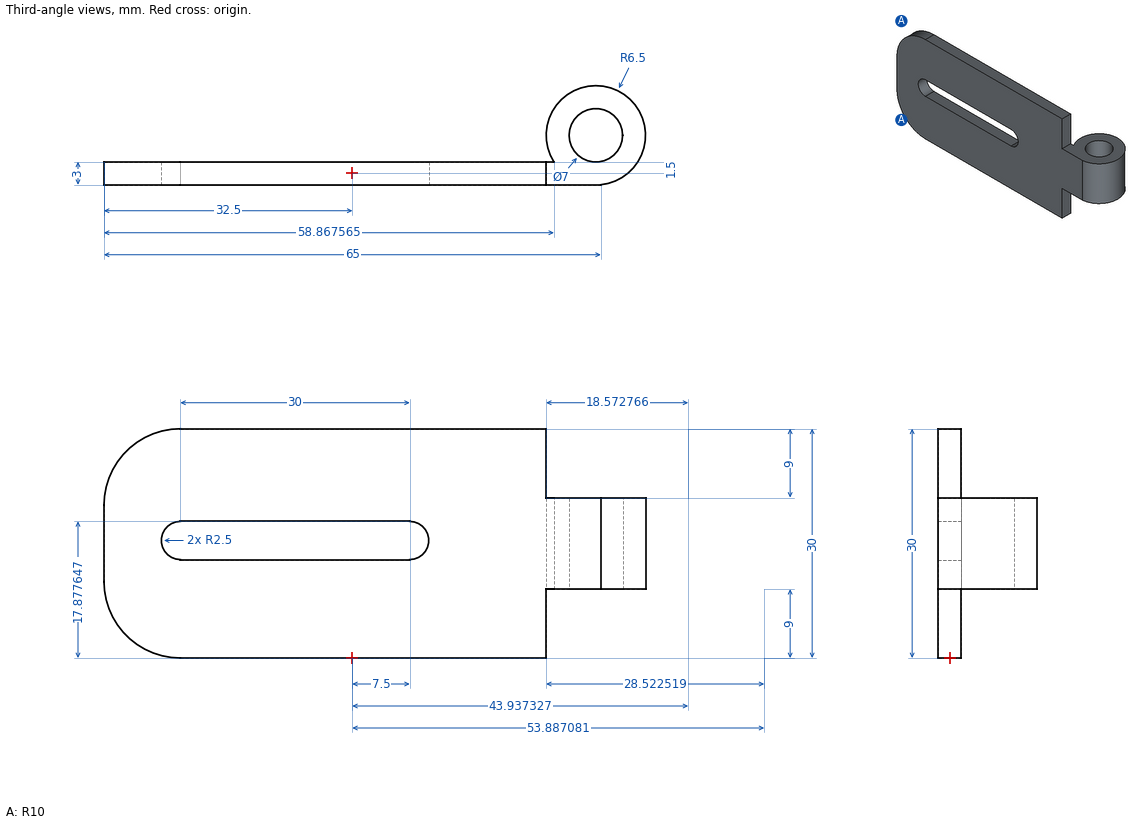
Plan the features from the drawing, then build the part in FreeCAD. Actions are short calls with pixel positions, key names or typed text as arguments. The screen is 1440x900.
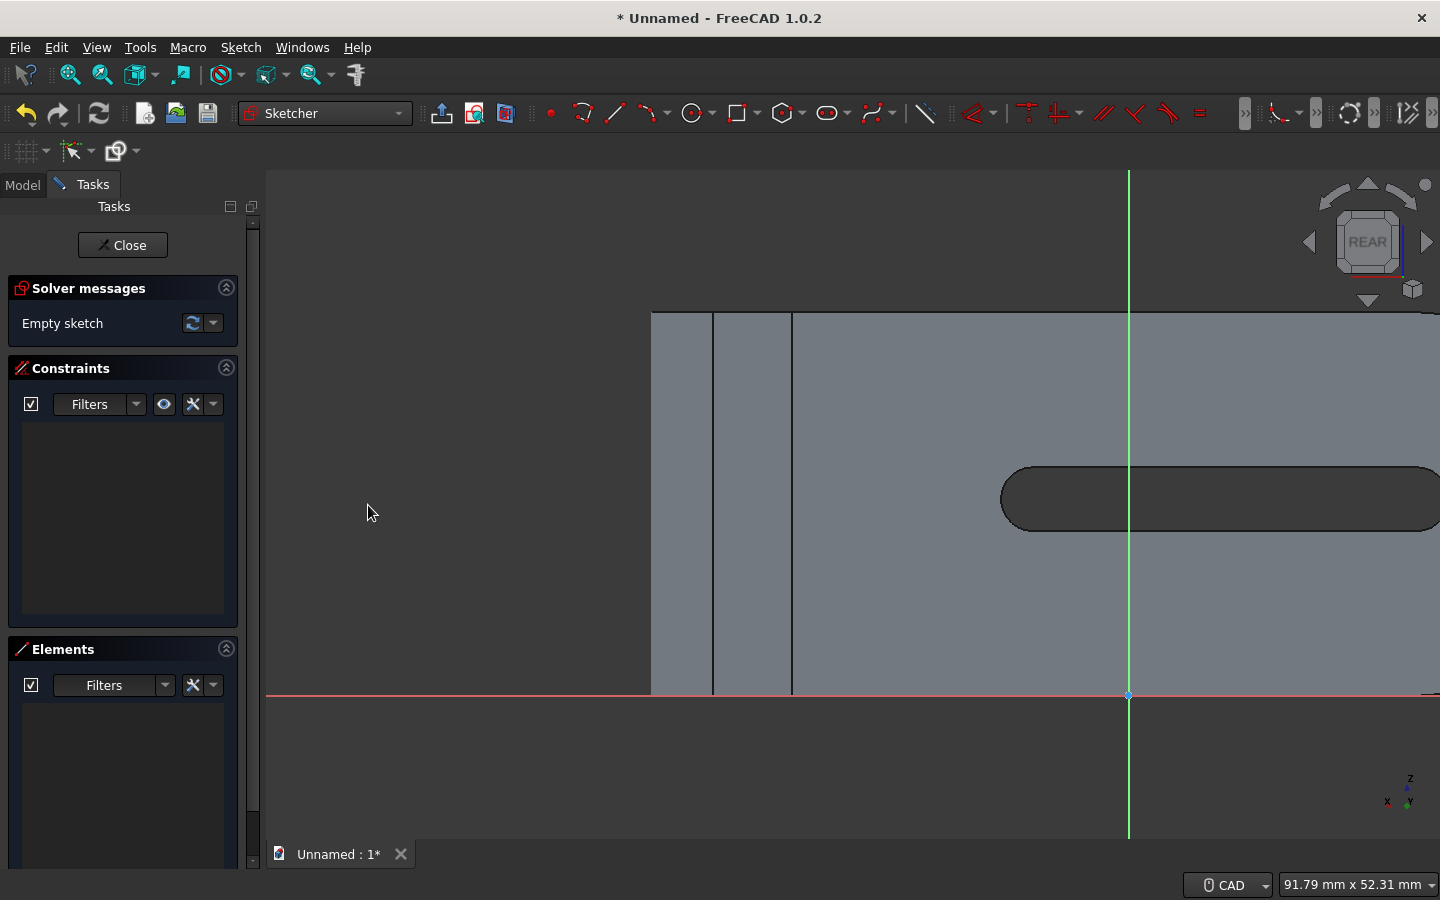
click(738, 114)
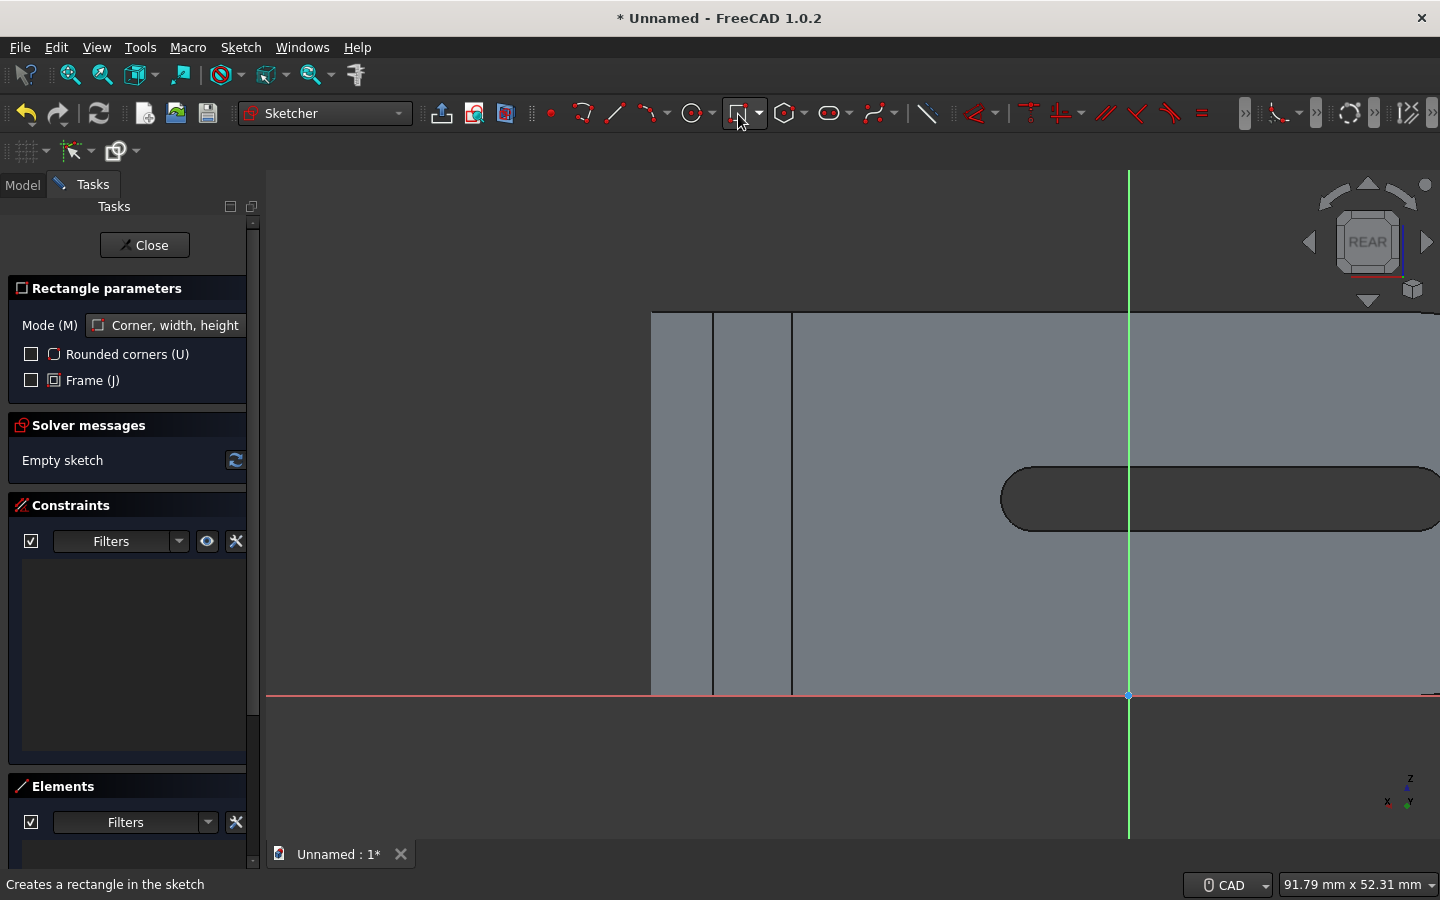
click(567, 312)
move(805, 427)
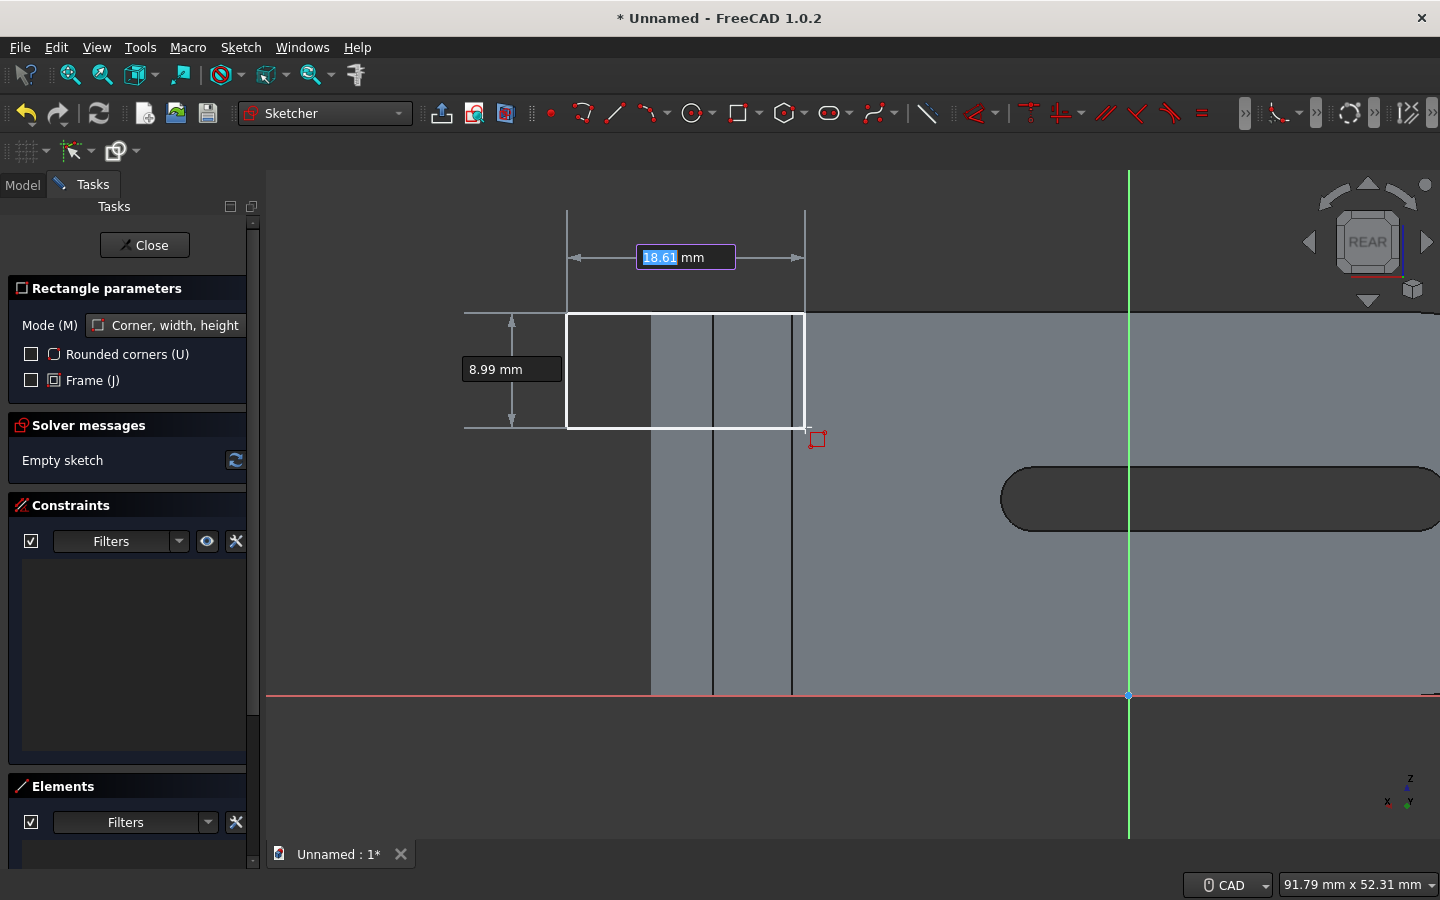
text(18.572766)
key(Tab)
text(9)
key(Return)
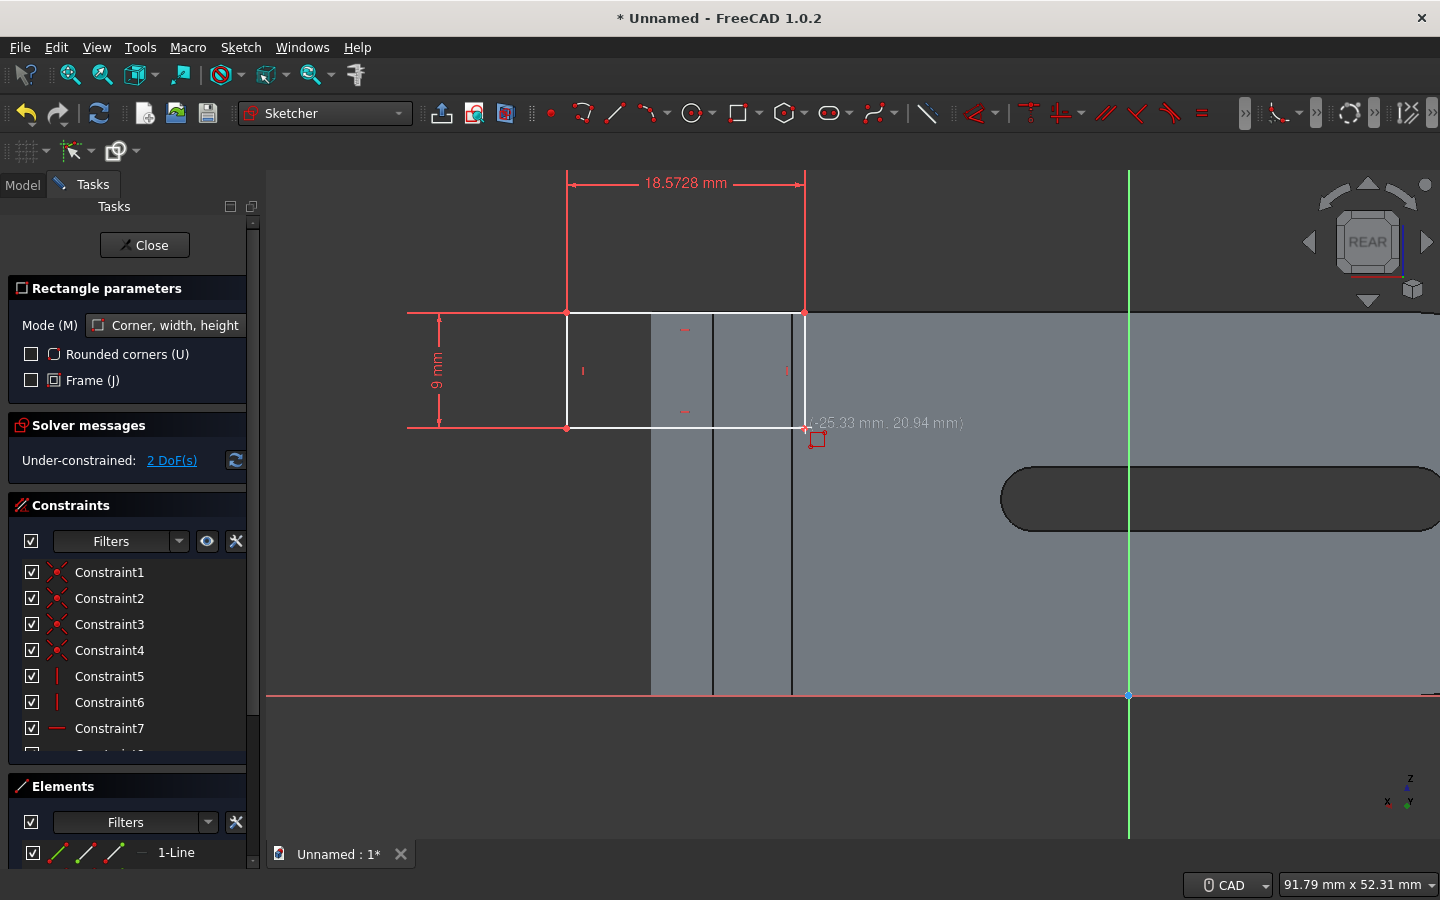
click(440, 581)
click(805, 696)
key(Escape)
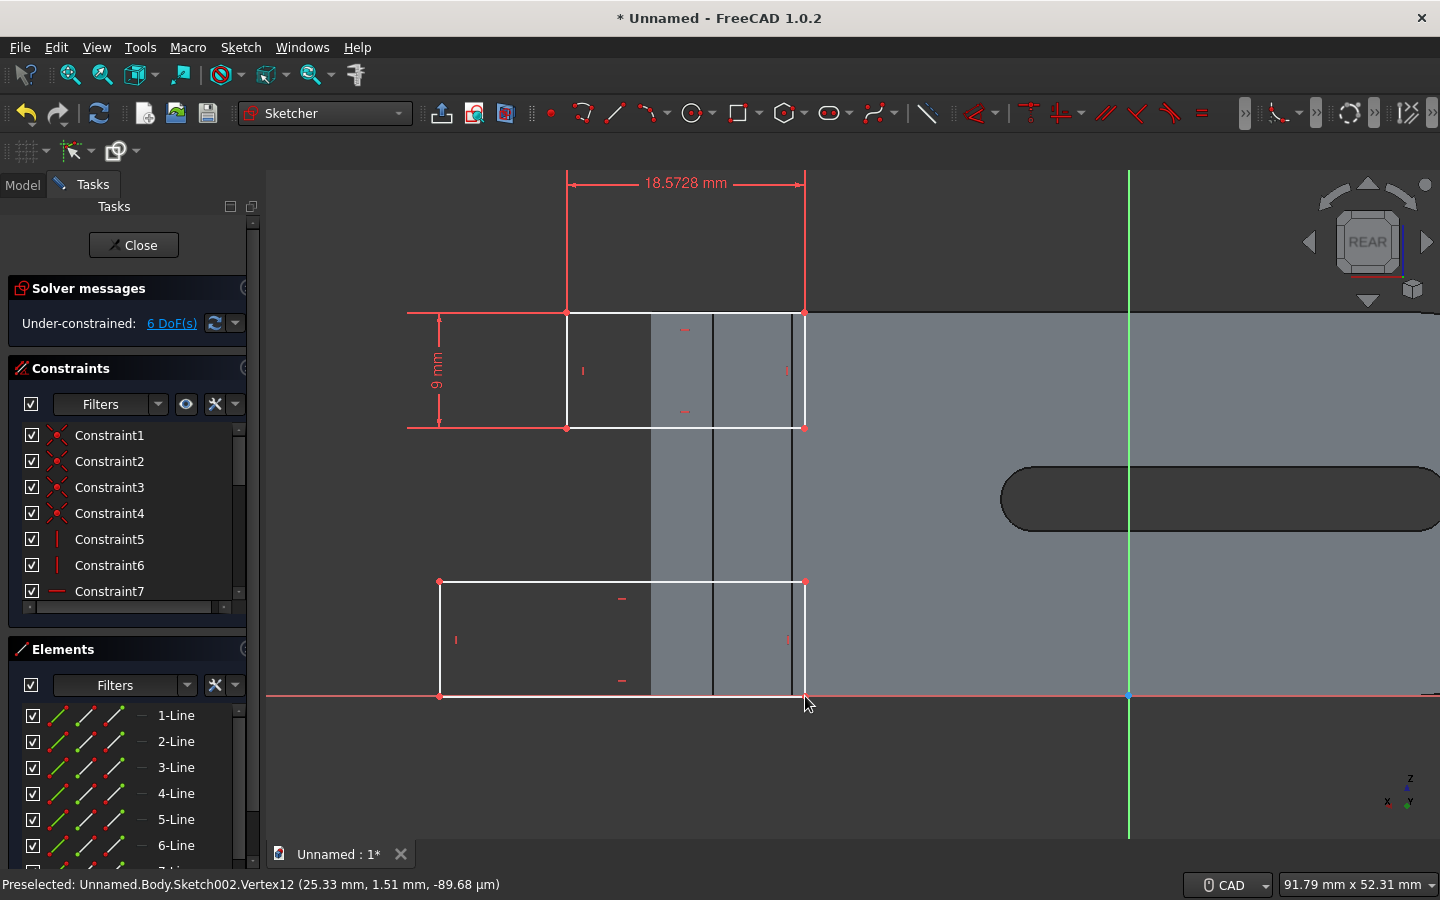
click(440, 697)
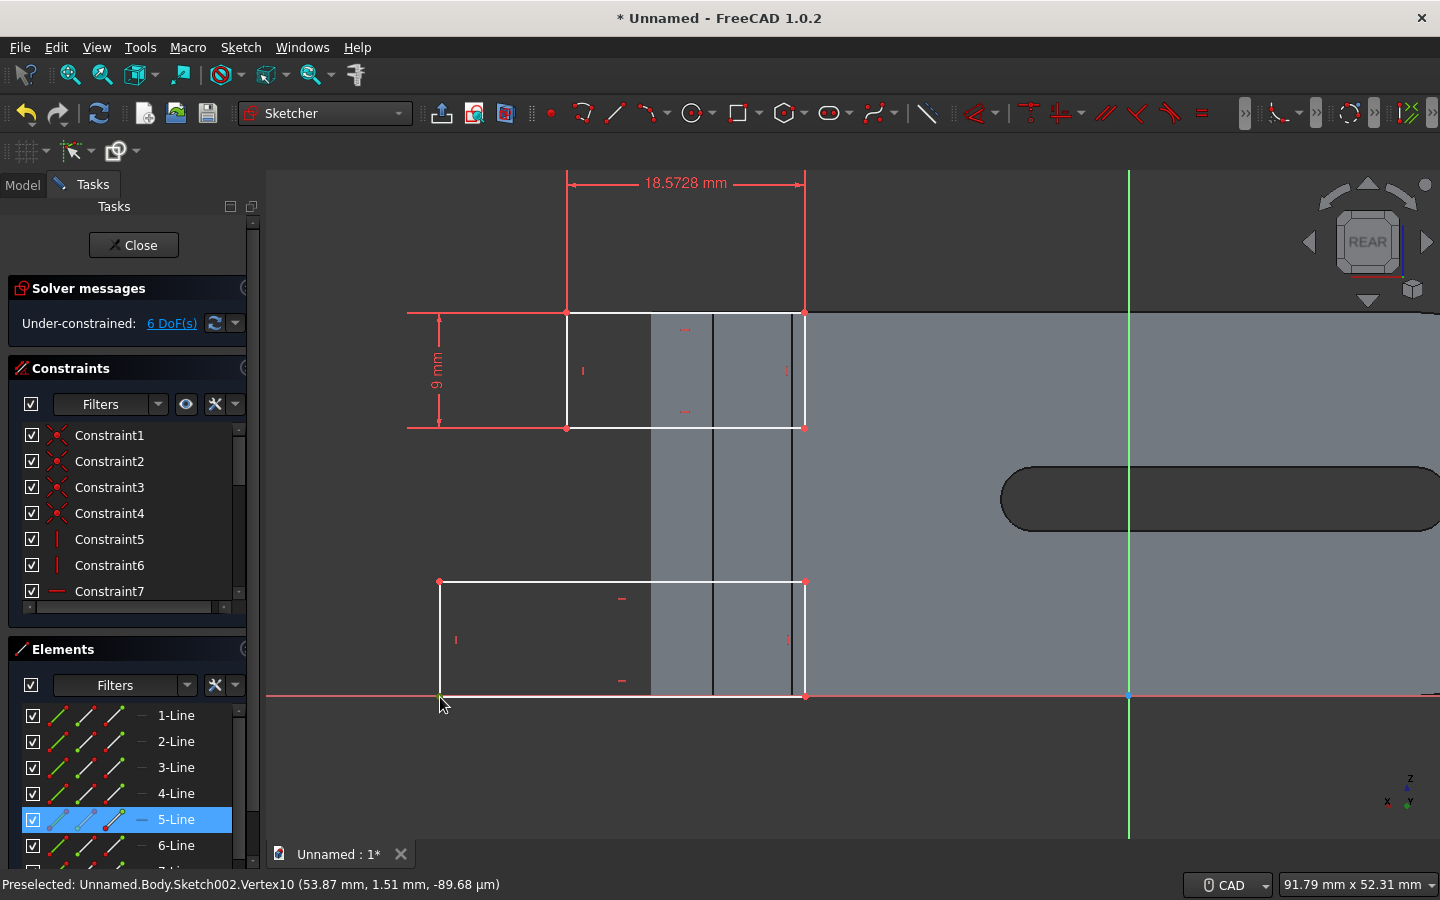
click(364, 696)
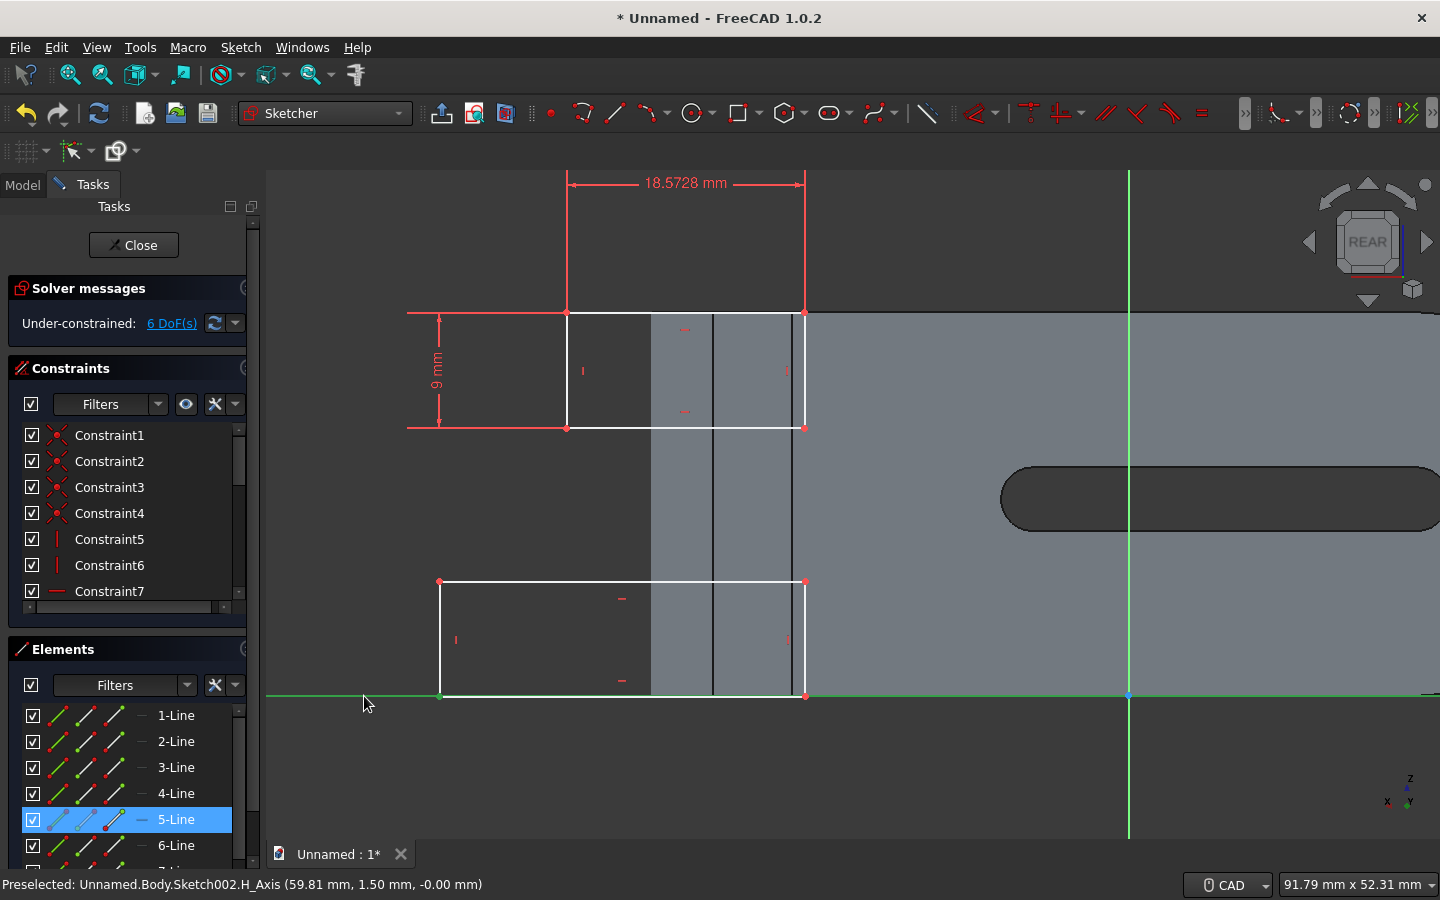
click(1030, 114)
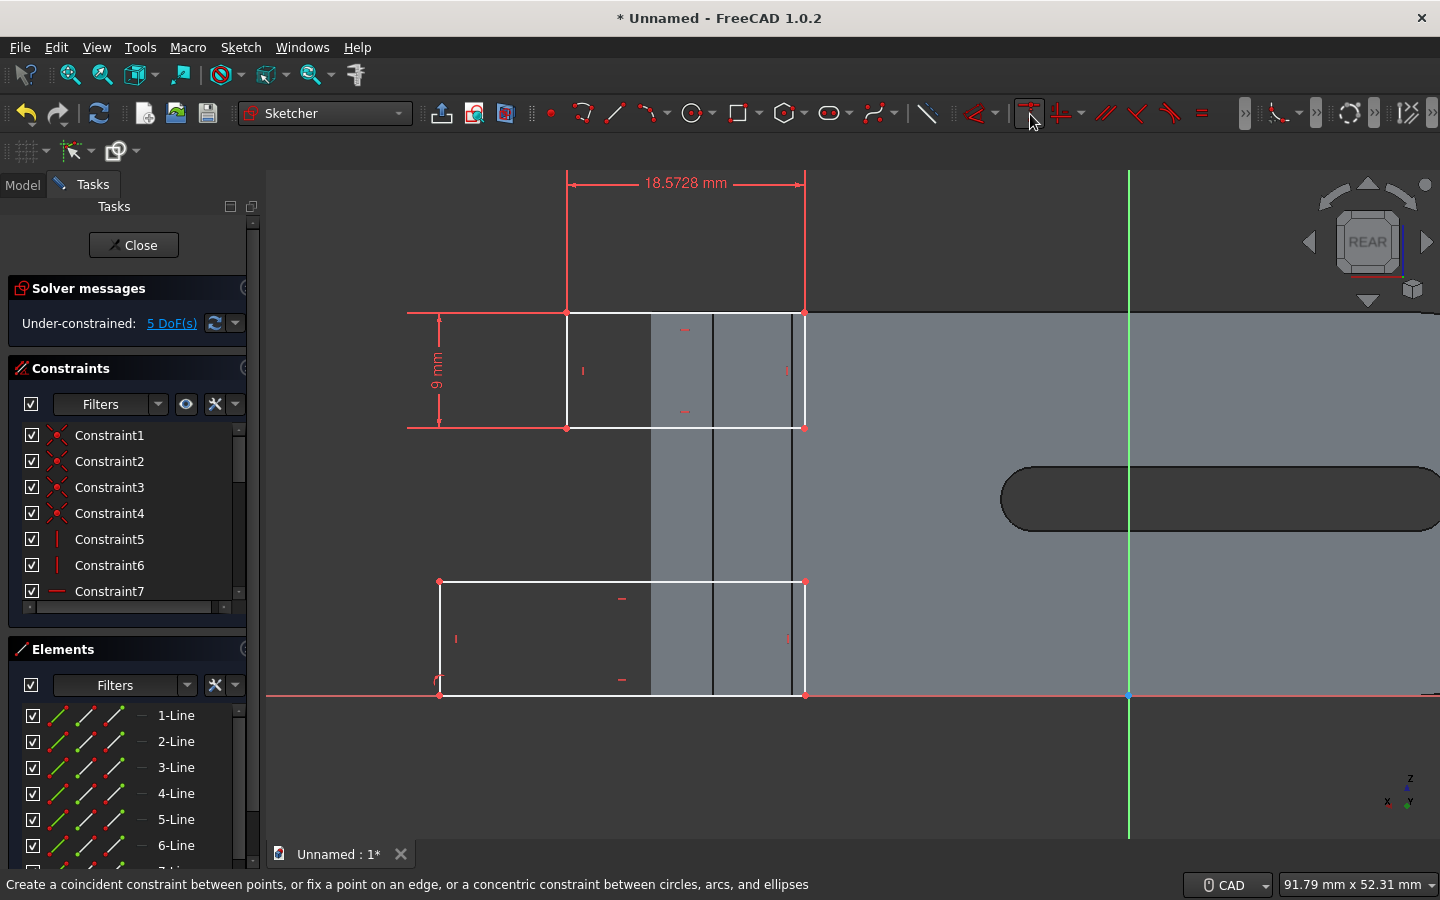
click(974, 114)